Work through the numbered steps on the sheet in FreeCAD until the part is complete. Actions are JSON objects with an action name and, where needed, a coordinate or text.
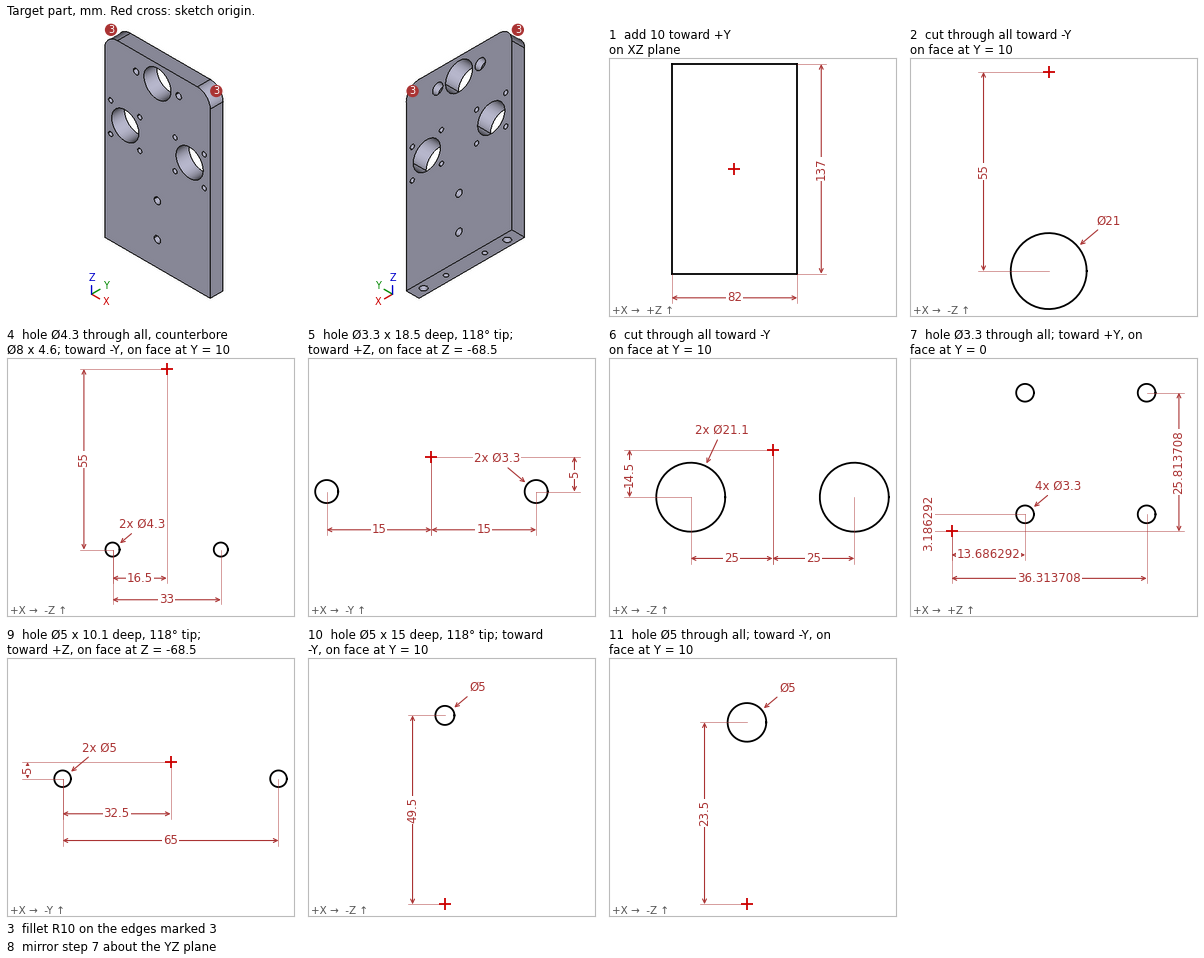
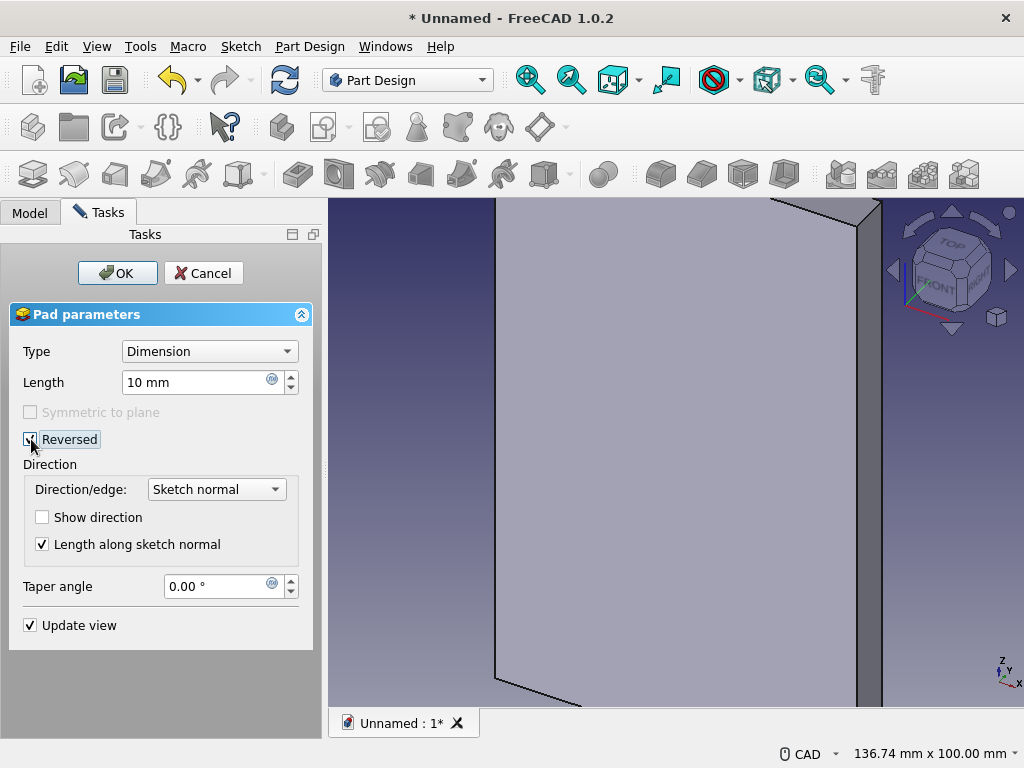
{"action": "left_click", "coordinate": [118, 273]}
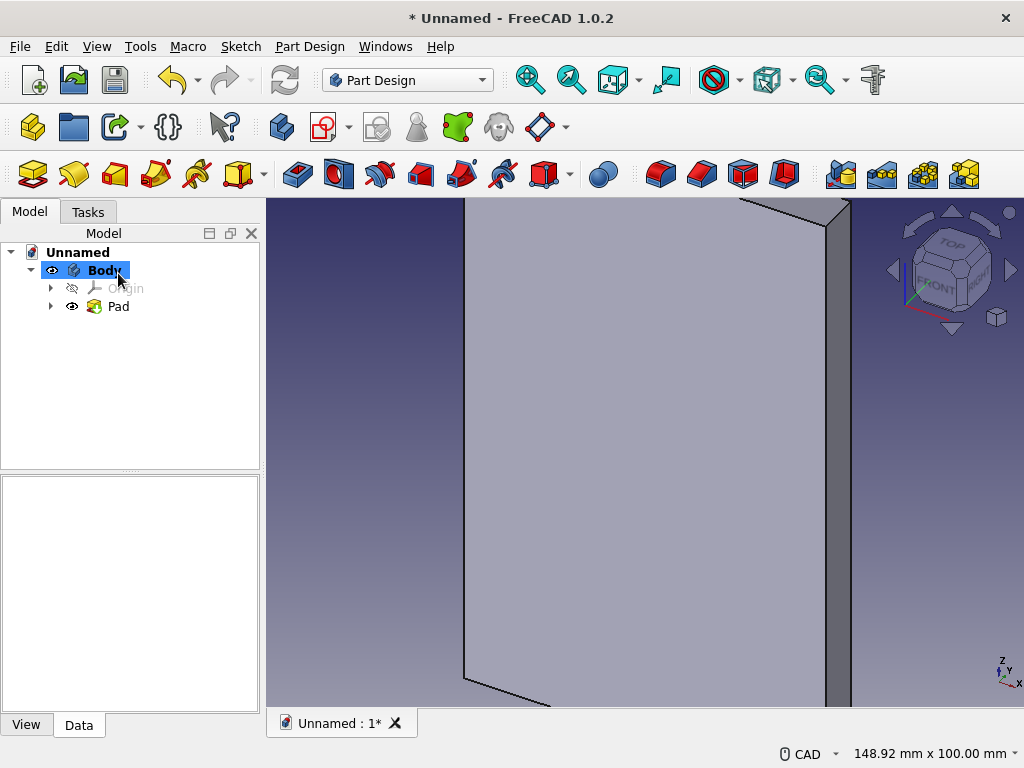
{"action": "key", "text": "v f"}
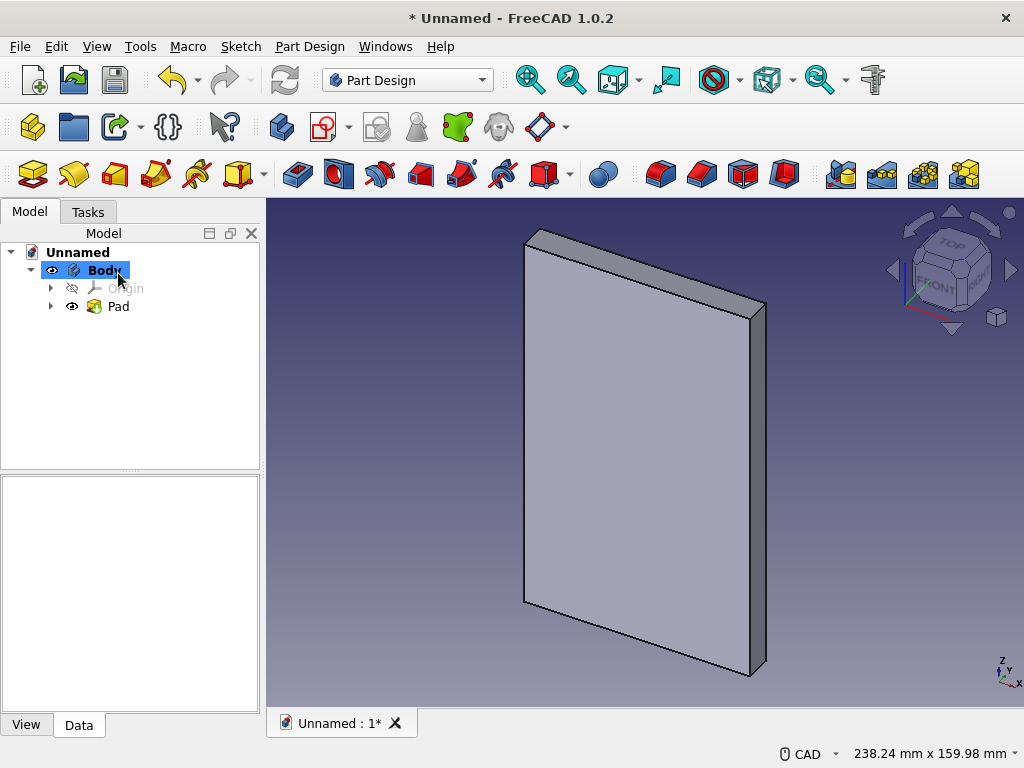
{"action": "key", "text": "4"}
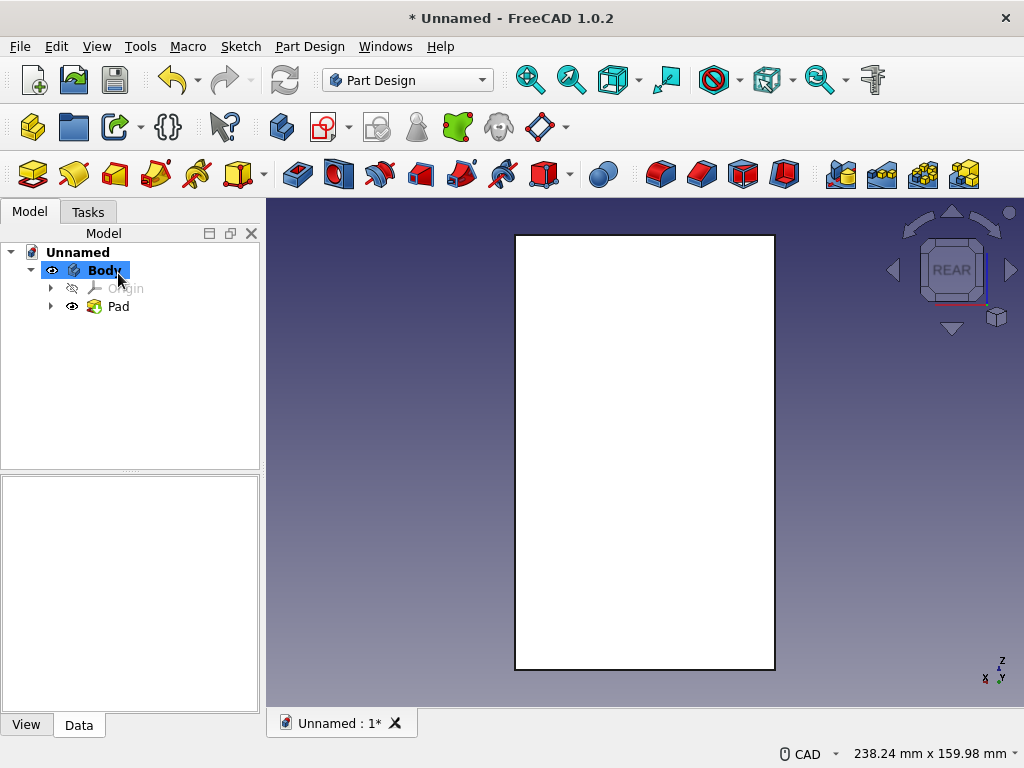
{"action": "left_click", "coordinate": [645, 389]}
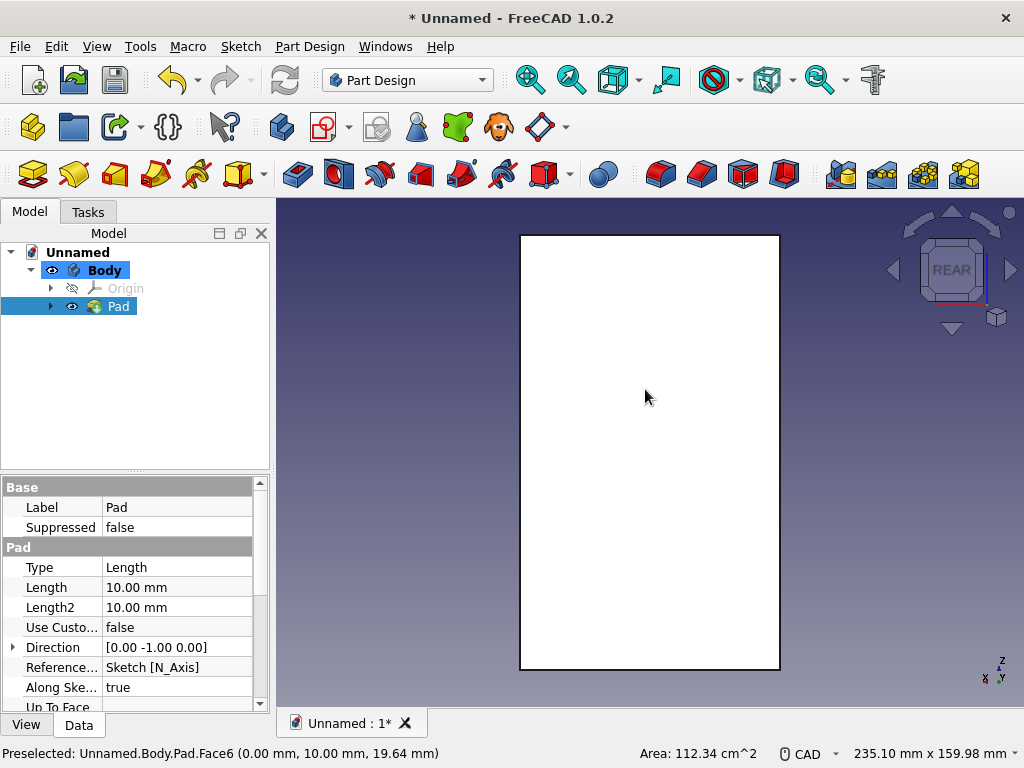
{"action": "left_click", "coordinate": [322, 128]}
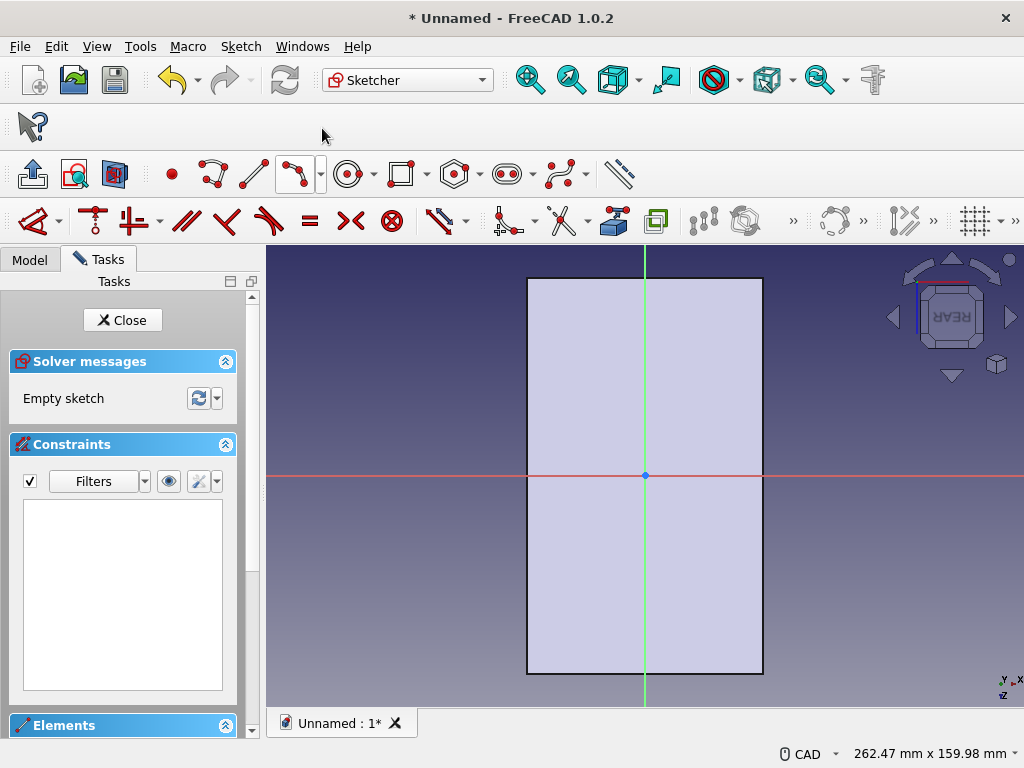
{"action": "scroll", "coordinate": [662, 675], "scroll_direction": "up", "scroll_amount": 8}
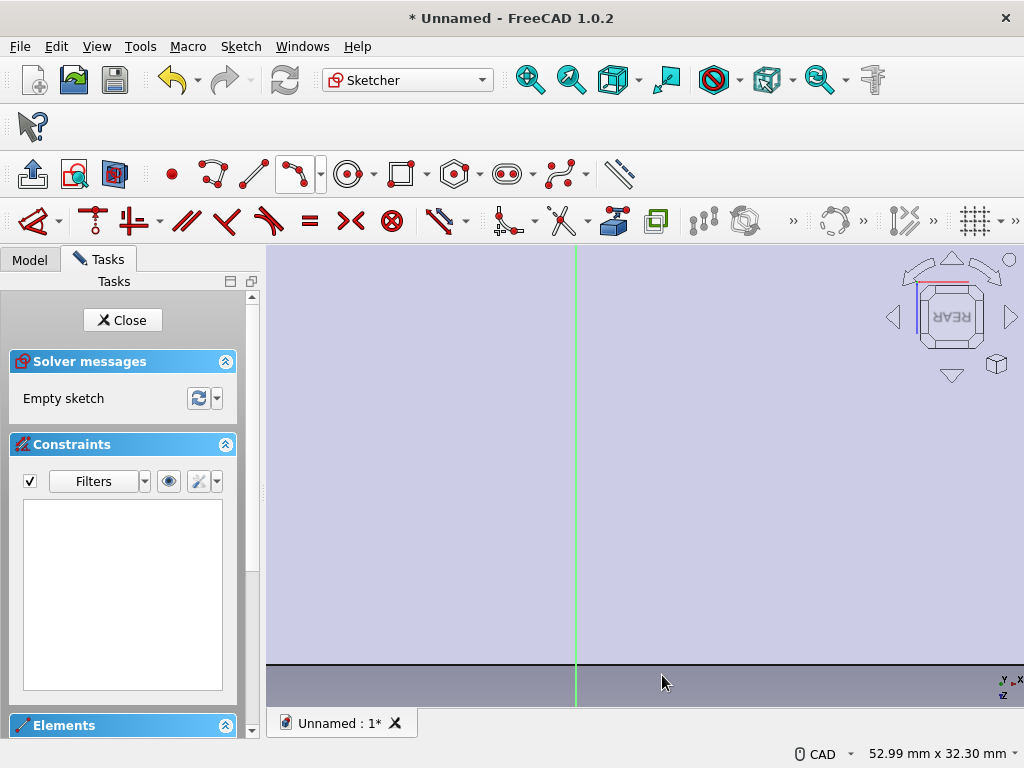
{"action": "key", "text": "g c"}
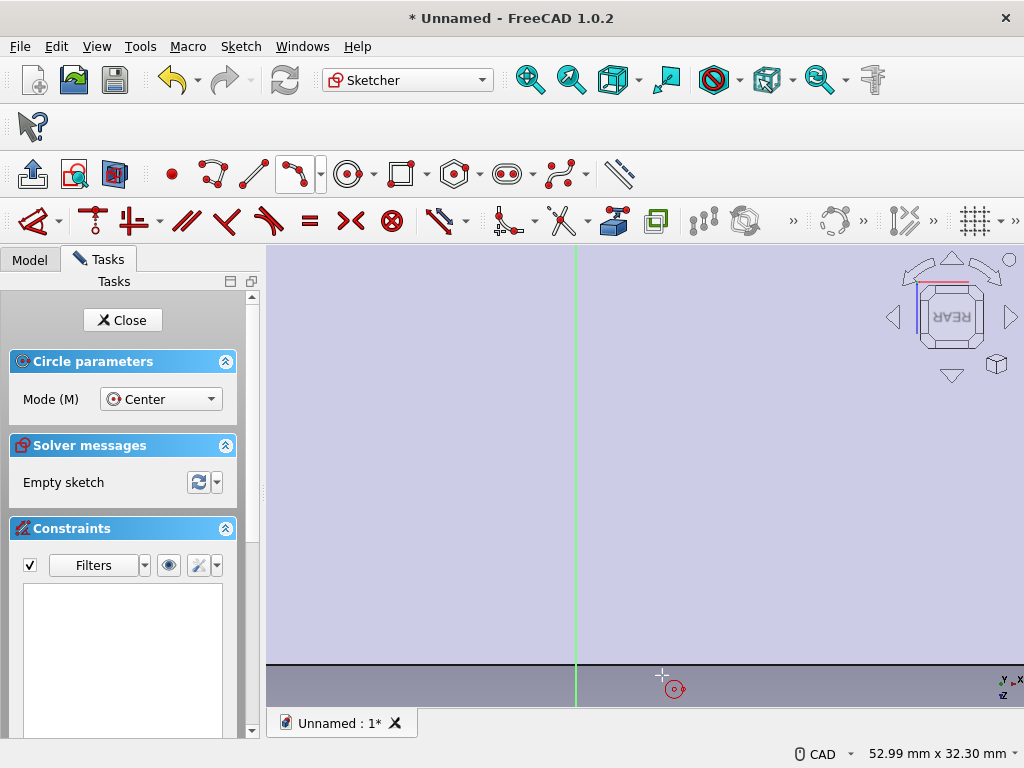
{"action": "left_click", "coordinate": [576, 472]}
{"action": "mouse_move", "coordinate": [682, 366]}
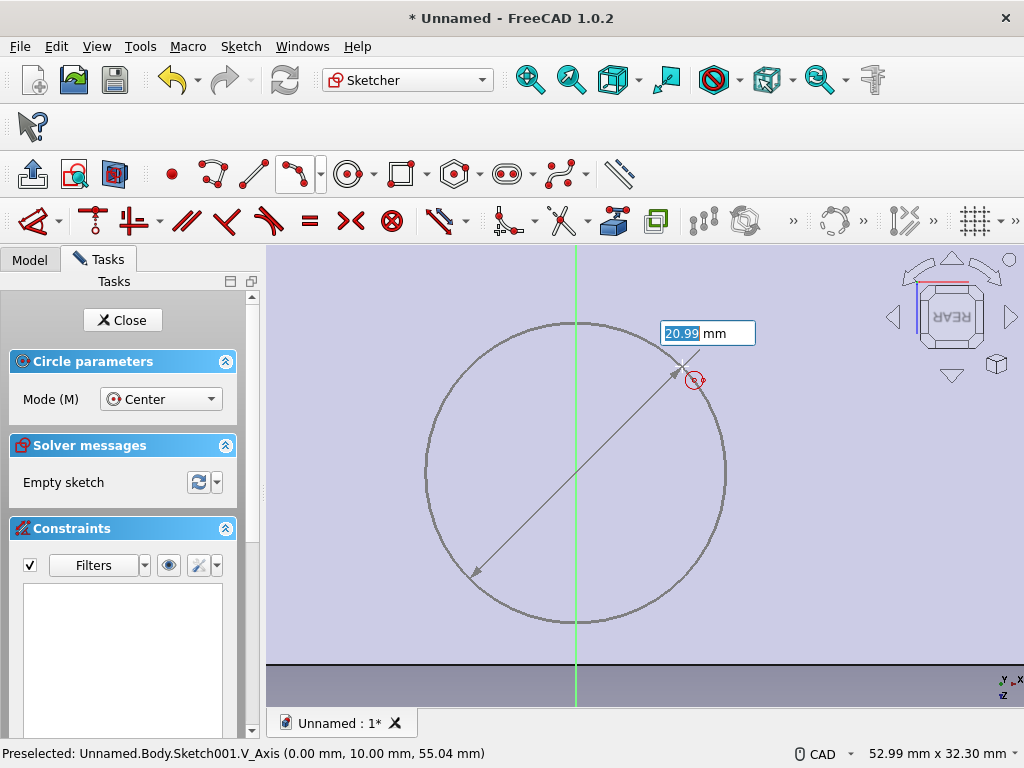
{"action": "type", "text": "21"}
{"action": "key", "text": "Return"}
{"action": "key", "text": "Escape"}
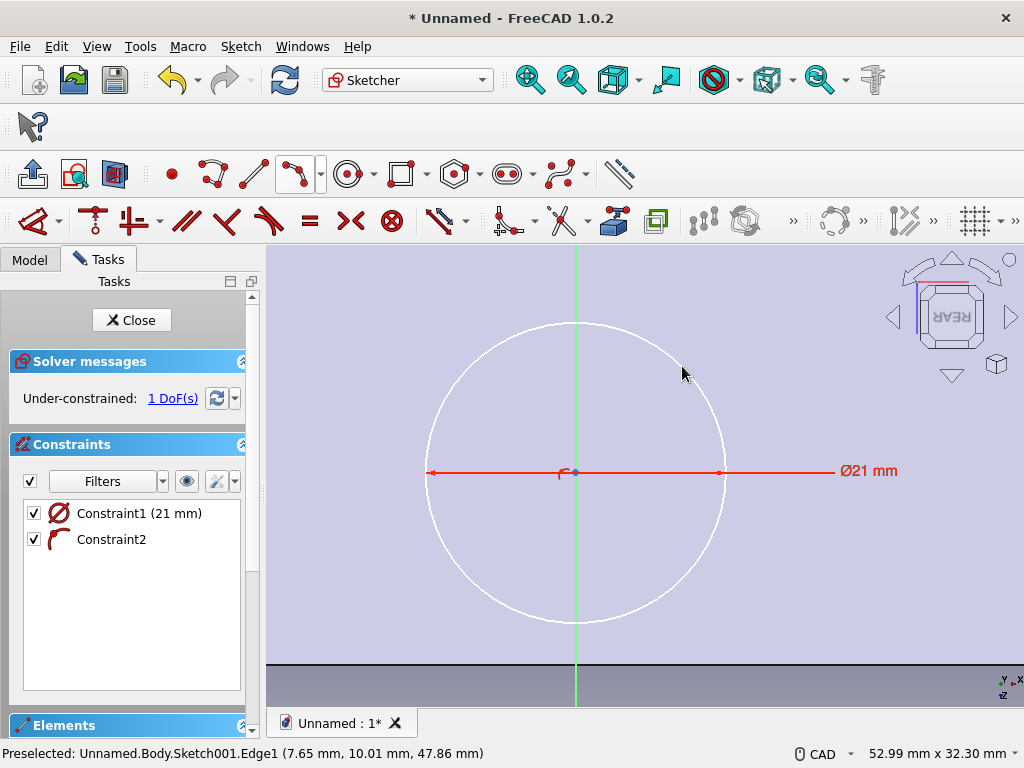
{"action": "left_click", "coordinate": [32, 222]}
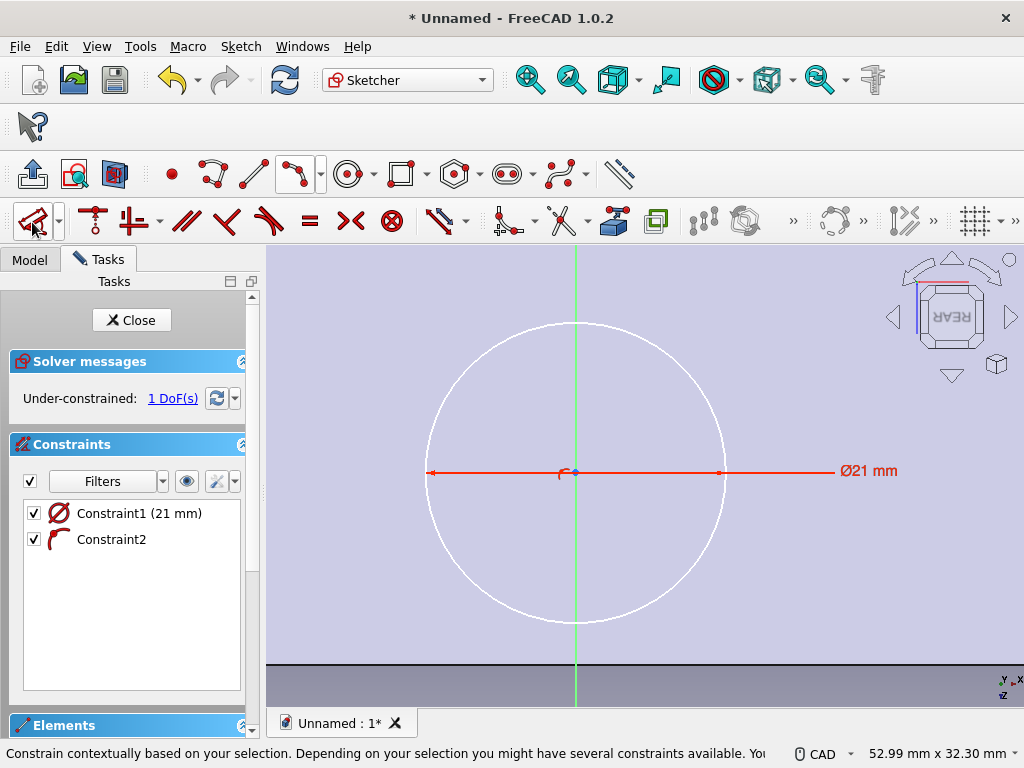
{"action": "left_click", "coordinate": [576, 473]}
{"action": "left_click", "coordinate": [610, 373]}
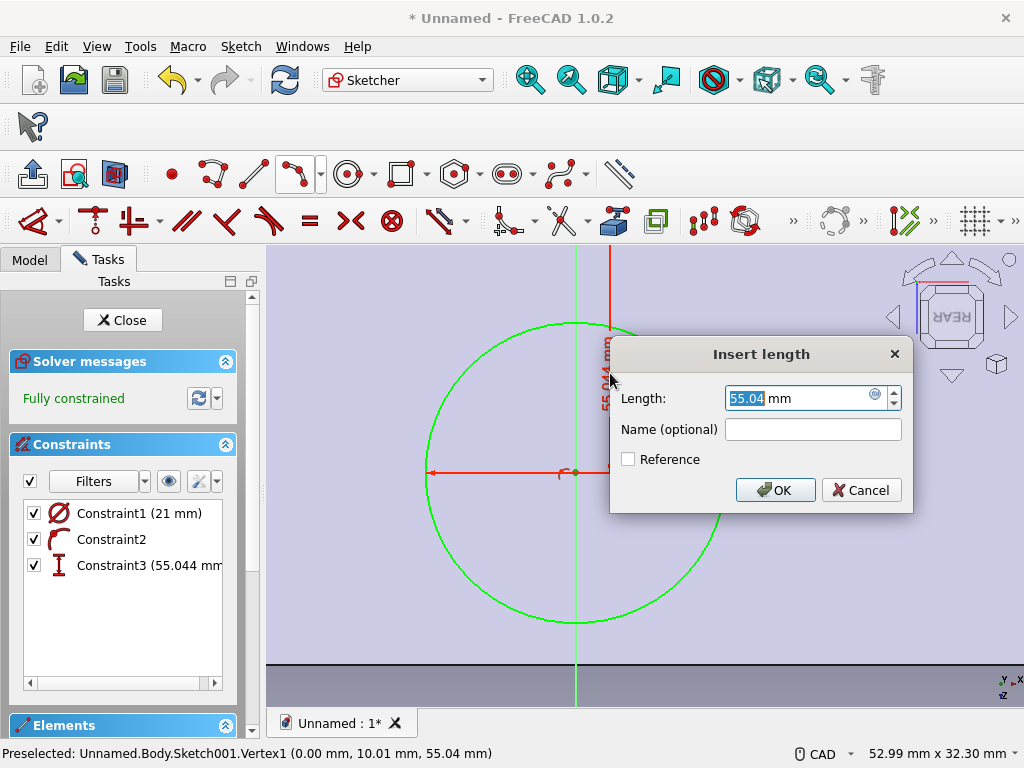
{"action": "type", "text": "55"}
{"action": "key", "text": "Return"}
{"action": "key", "text": "Escape"}